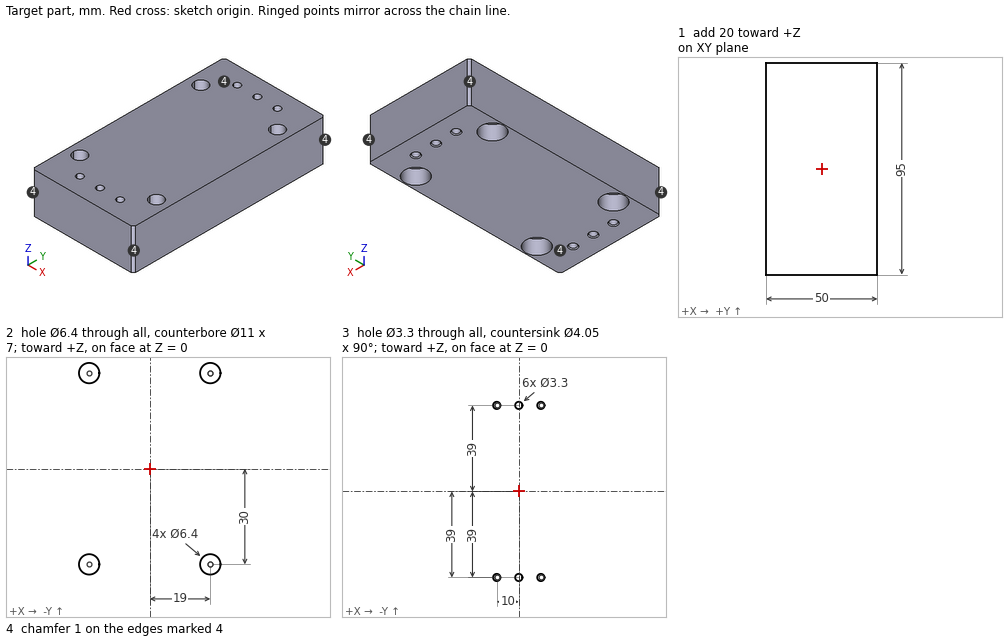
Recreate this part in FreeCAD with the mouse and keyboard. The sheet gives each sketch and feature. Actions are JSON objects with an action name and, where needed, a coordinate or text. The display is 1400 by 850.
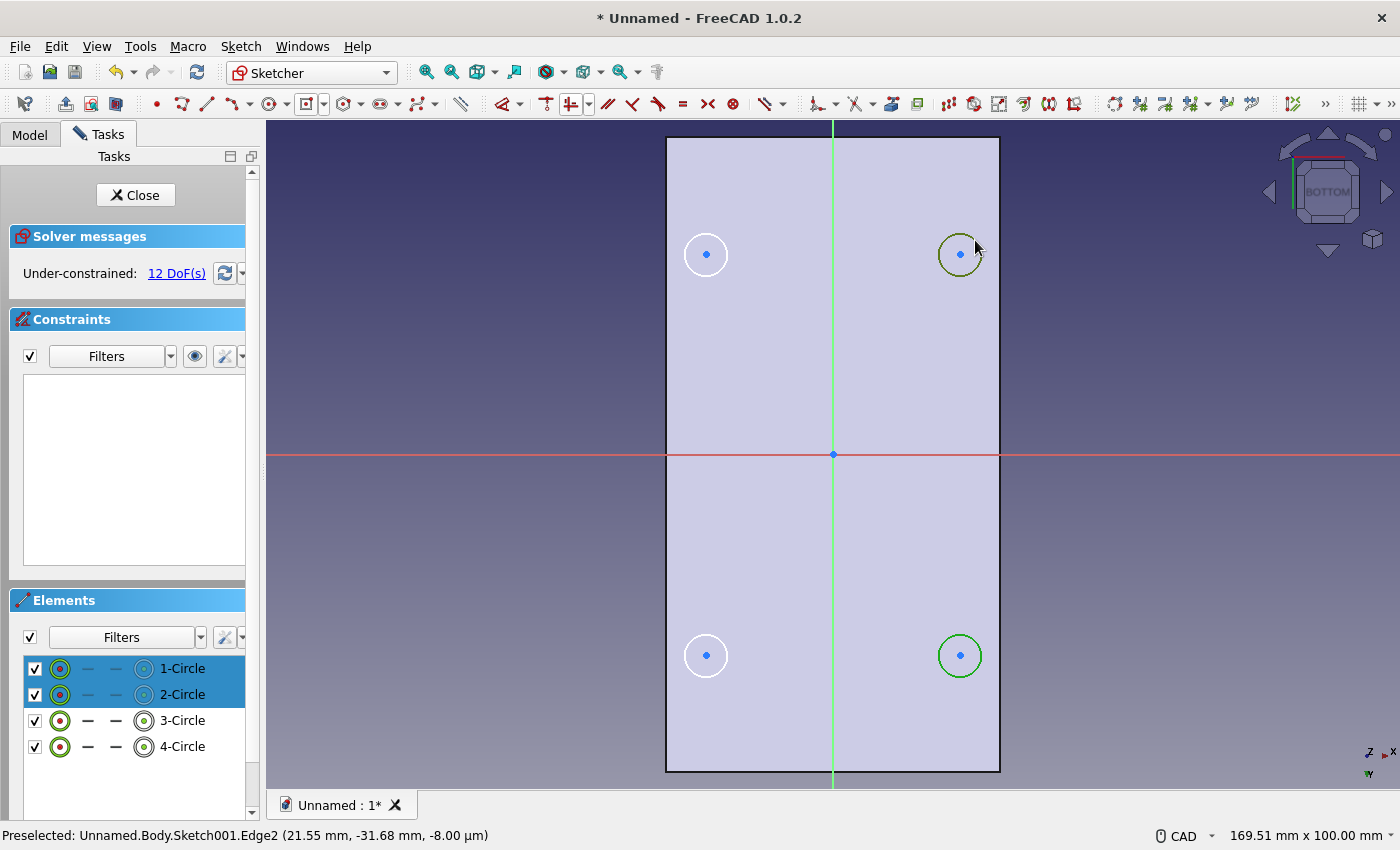
{"action": "left_click", "coordinate": [721, 240]}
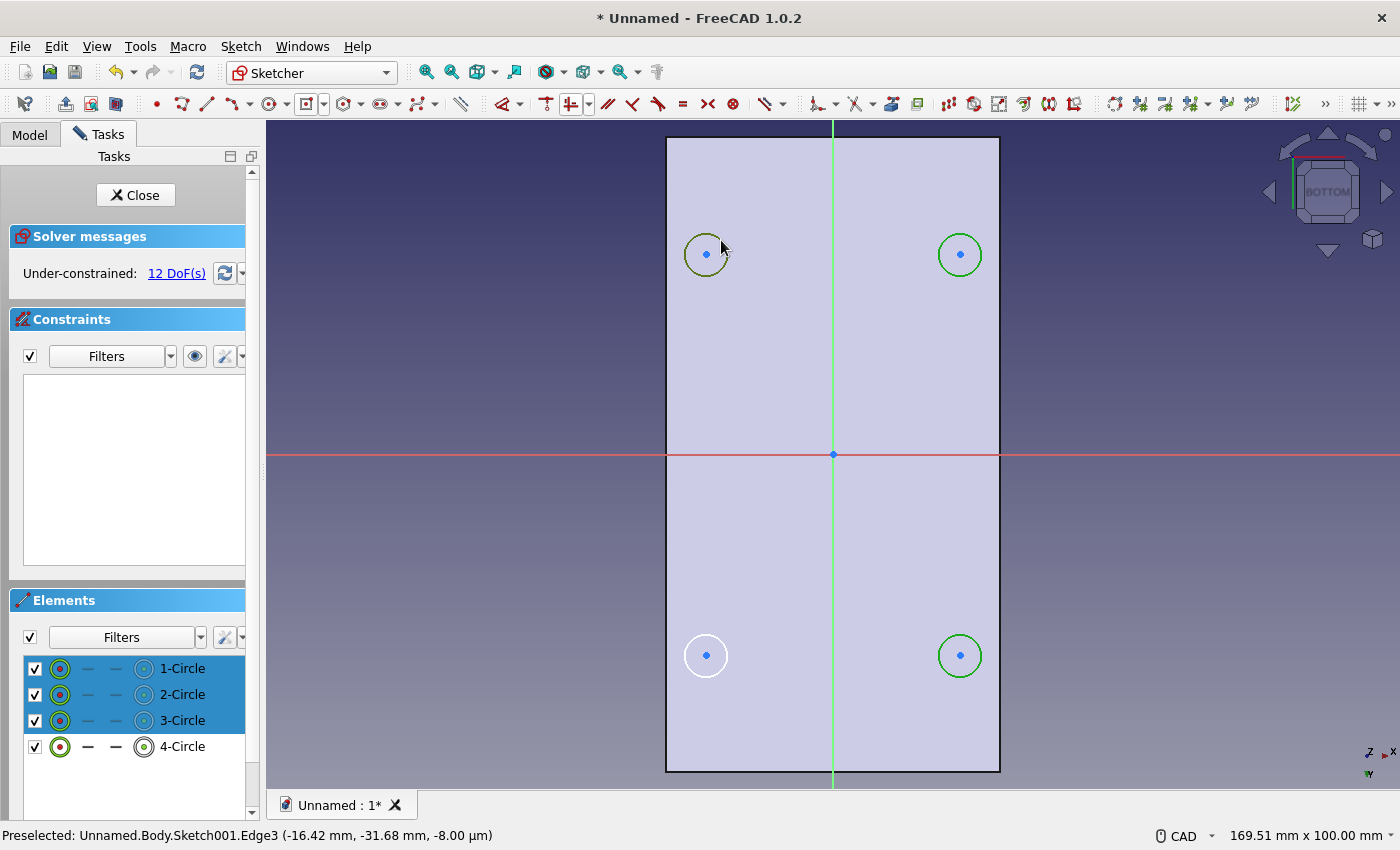
{"action": "left_click", "coordinate": [721, 641]}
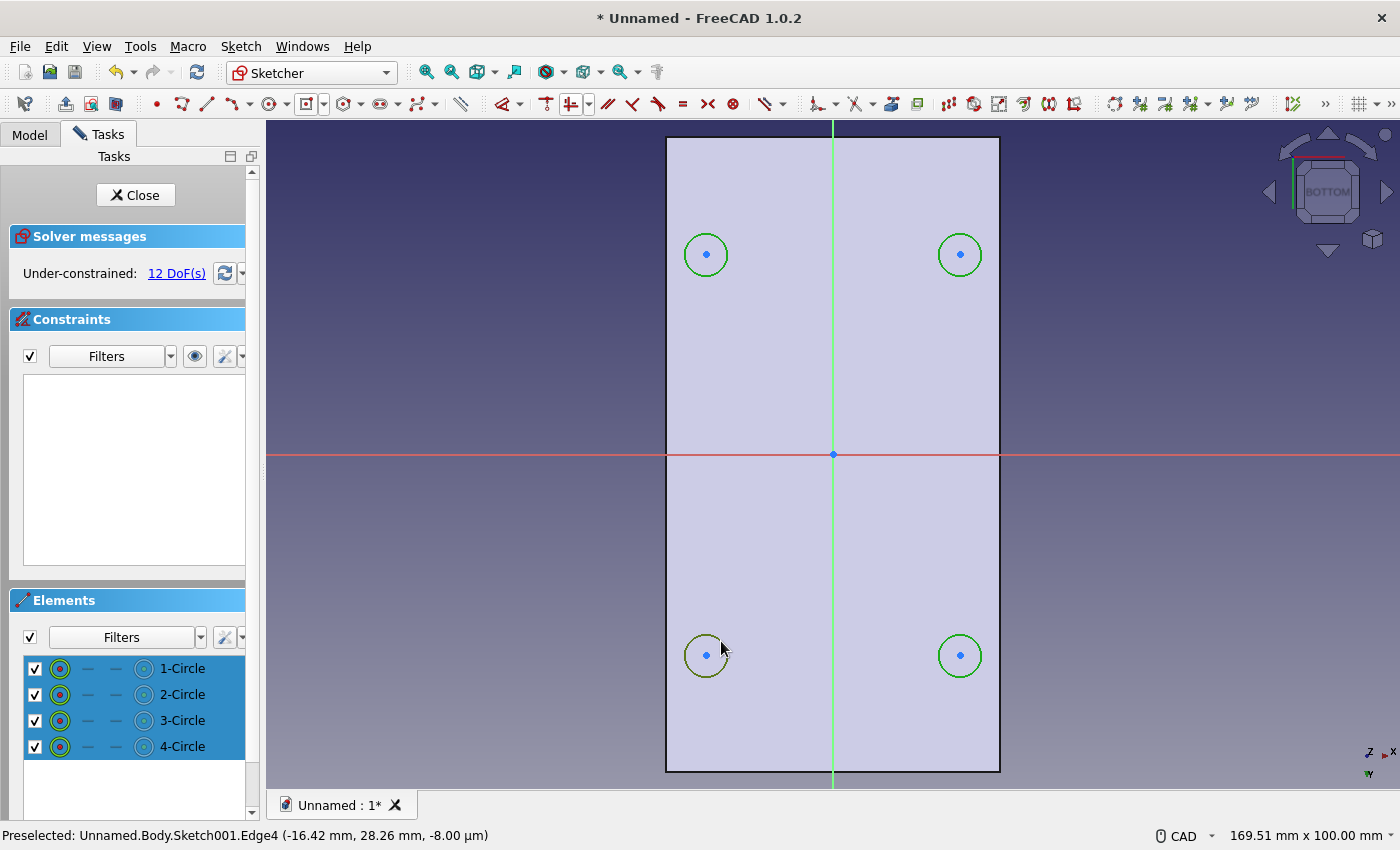
{"action": "key", "text": "e"}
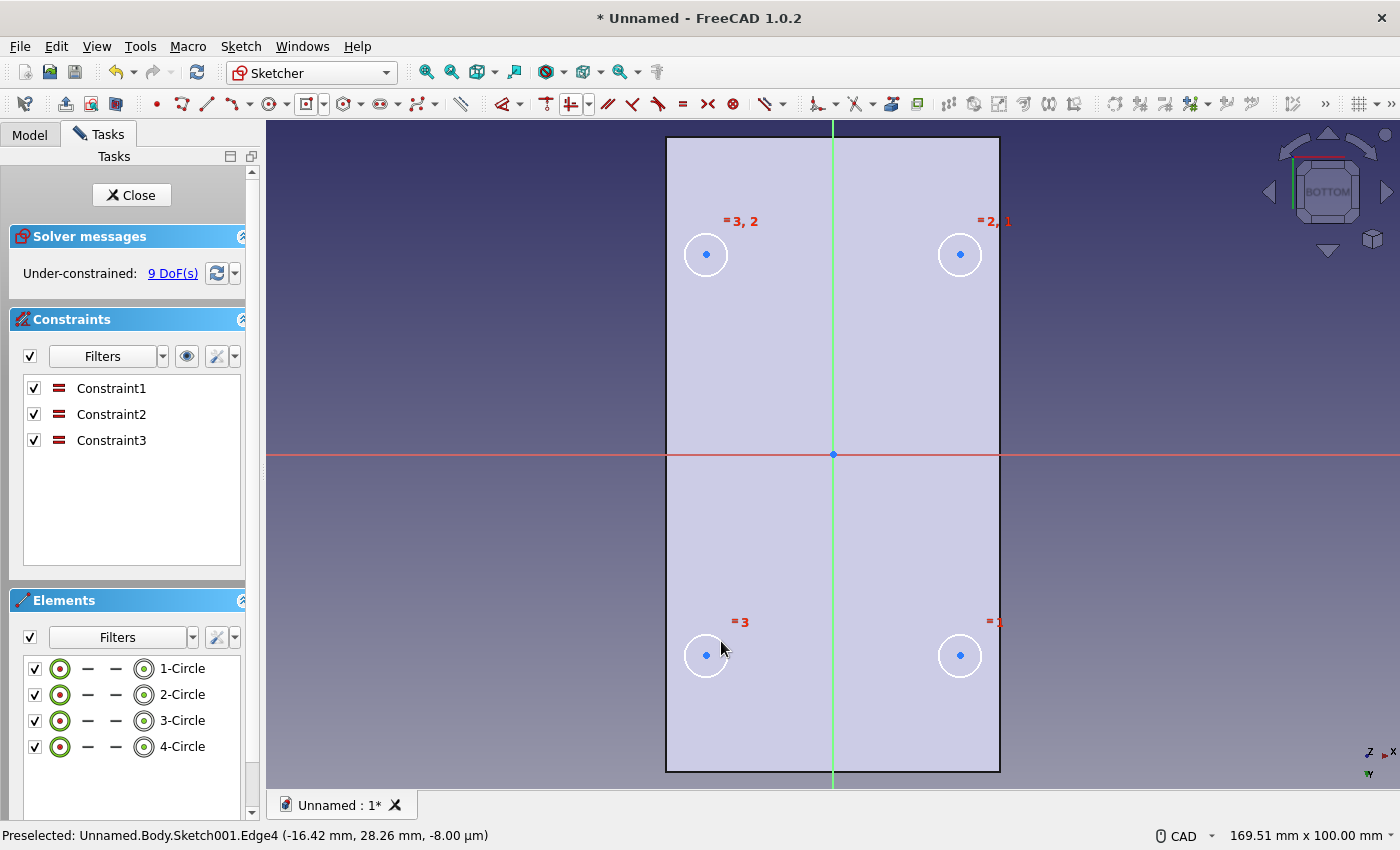
{"action": "left_click", "coordinate": [960, 656]}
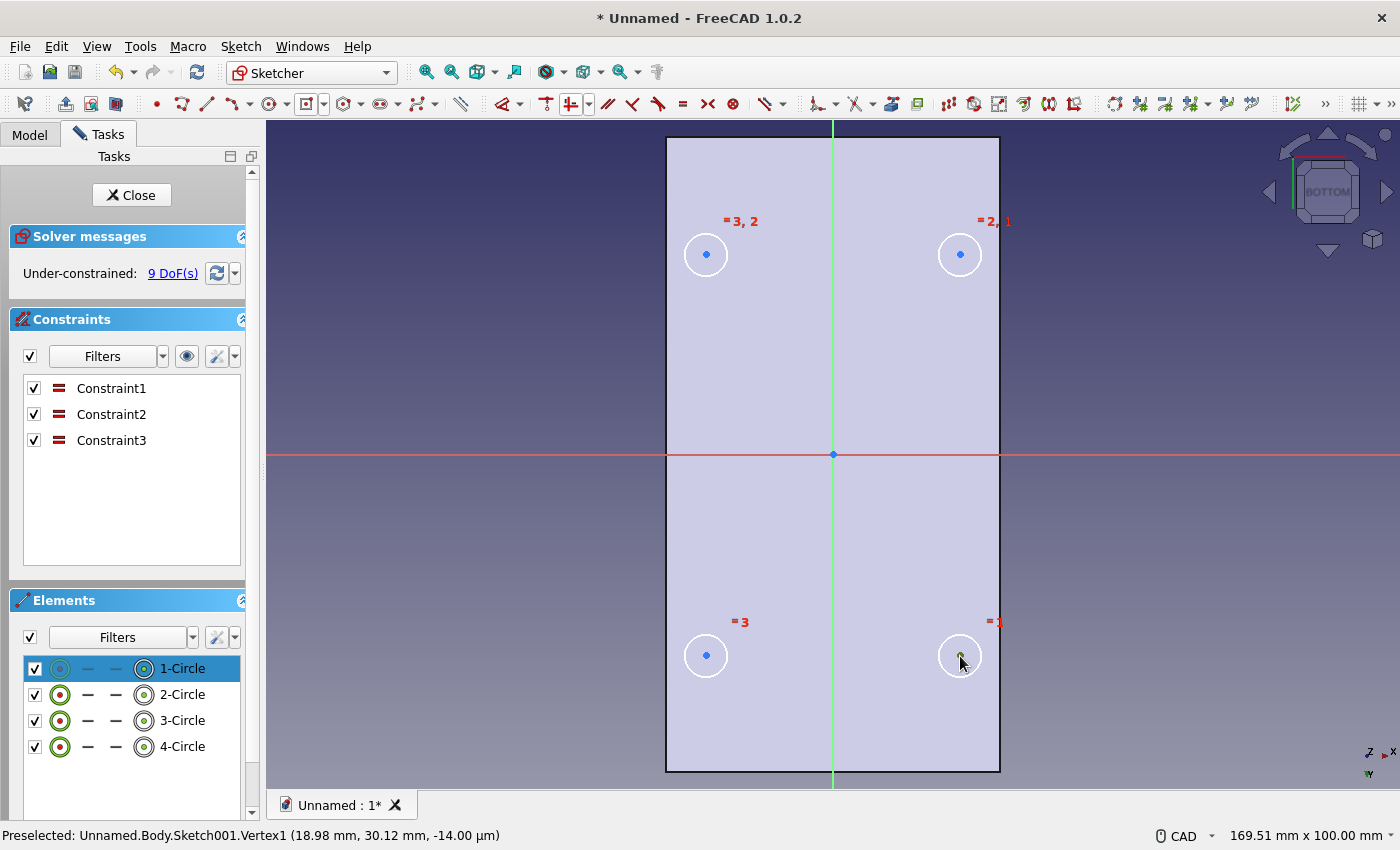
{"action": "left_click", "coordinate": [960, 255]}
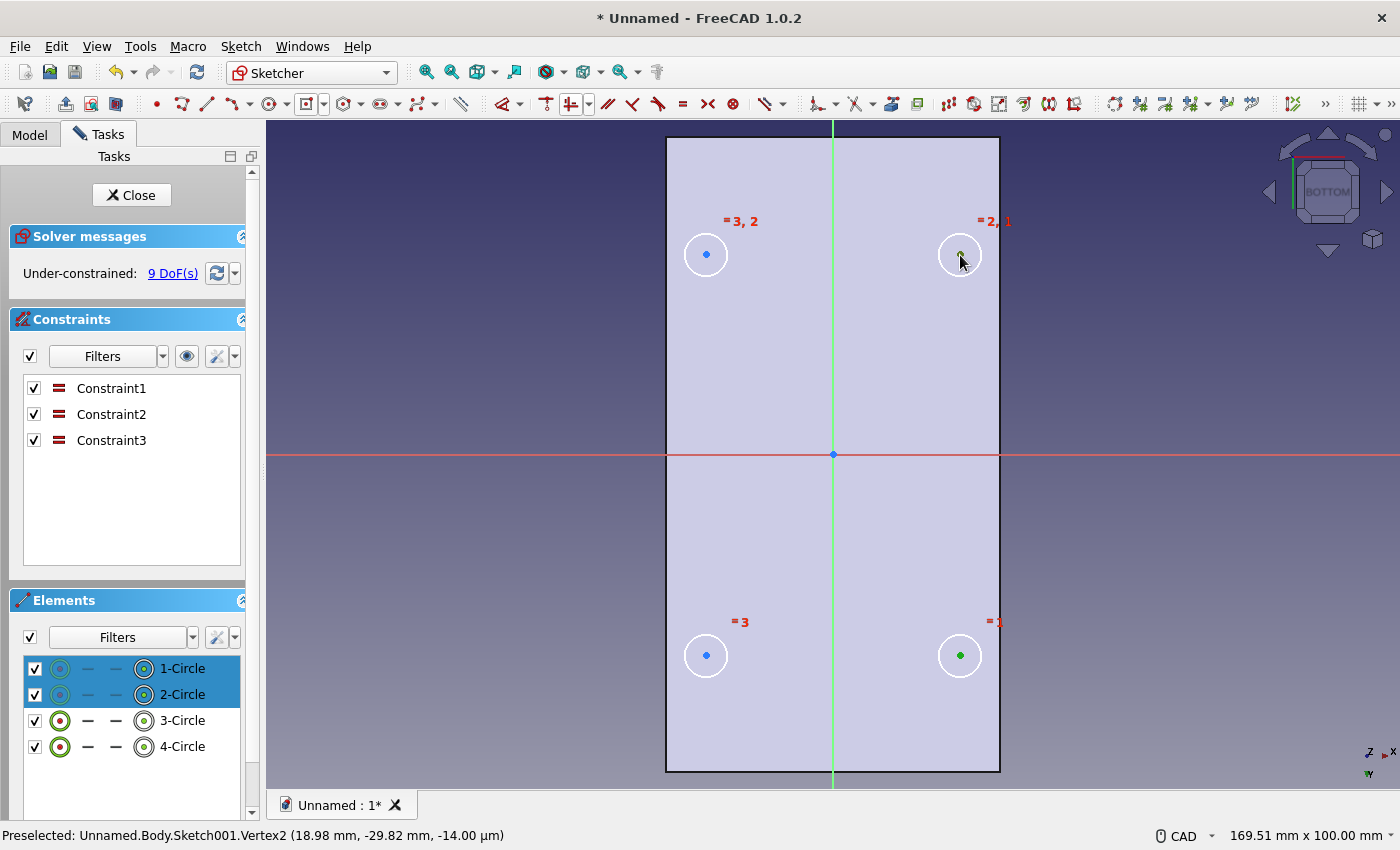
{"action": "left_click", "coordinate": [361, 454]}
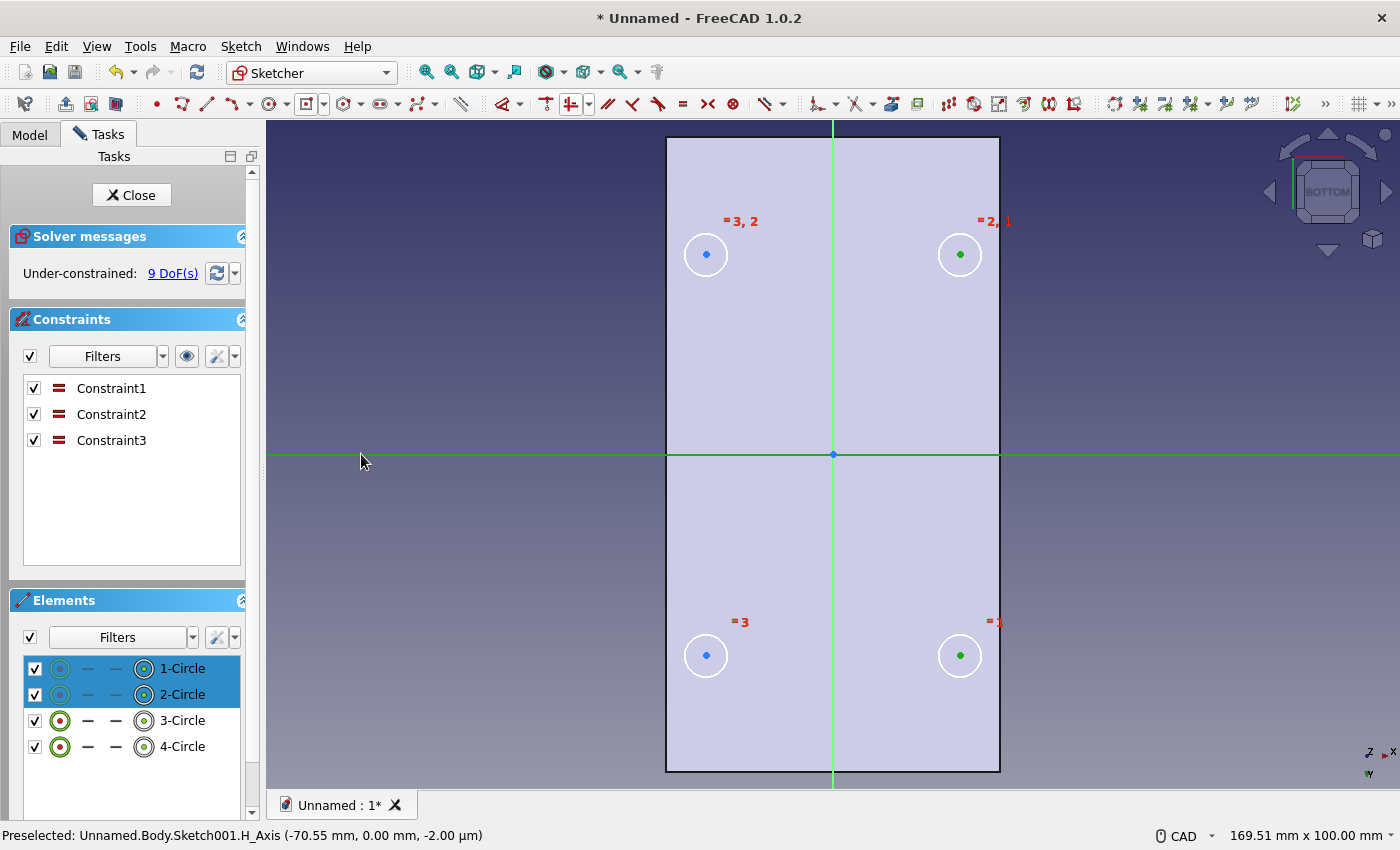
{"action": "left_click", "coordinate": [708, 104]}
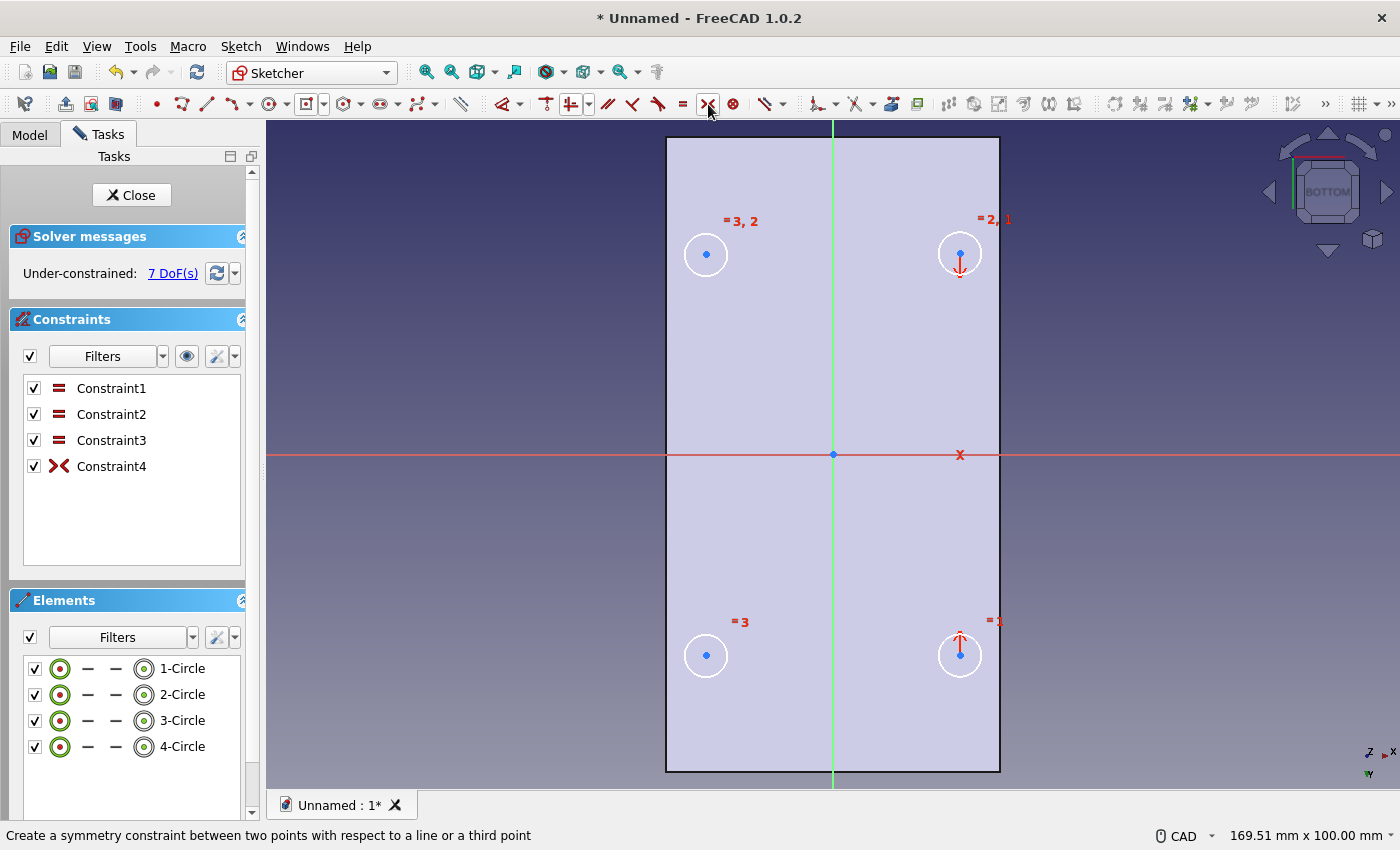
{"action": "left_click", "coordinate": [960, 253]}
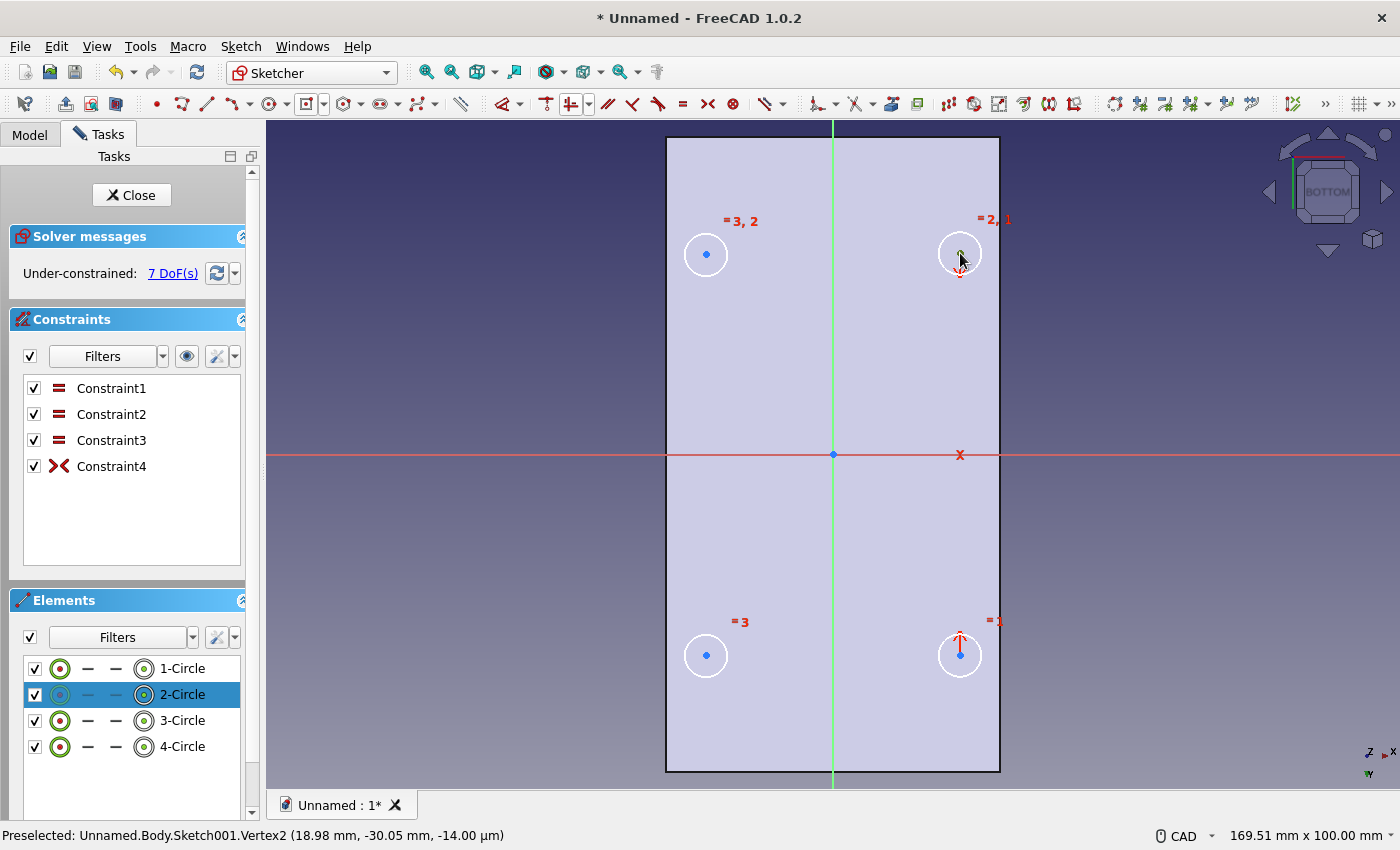
{"action": "left_click", "coordinate": [706, 255]}